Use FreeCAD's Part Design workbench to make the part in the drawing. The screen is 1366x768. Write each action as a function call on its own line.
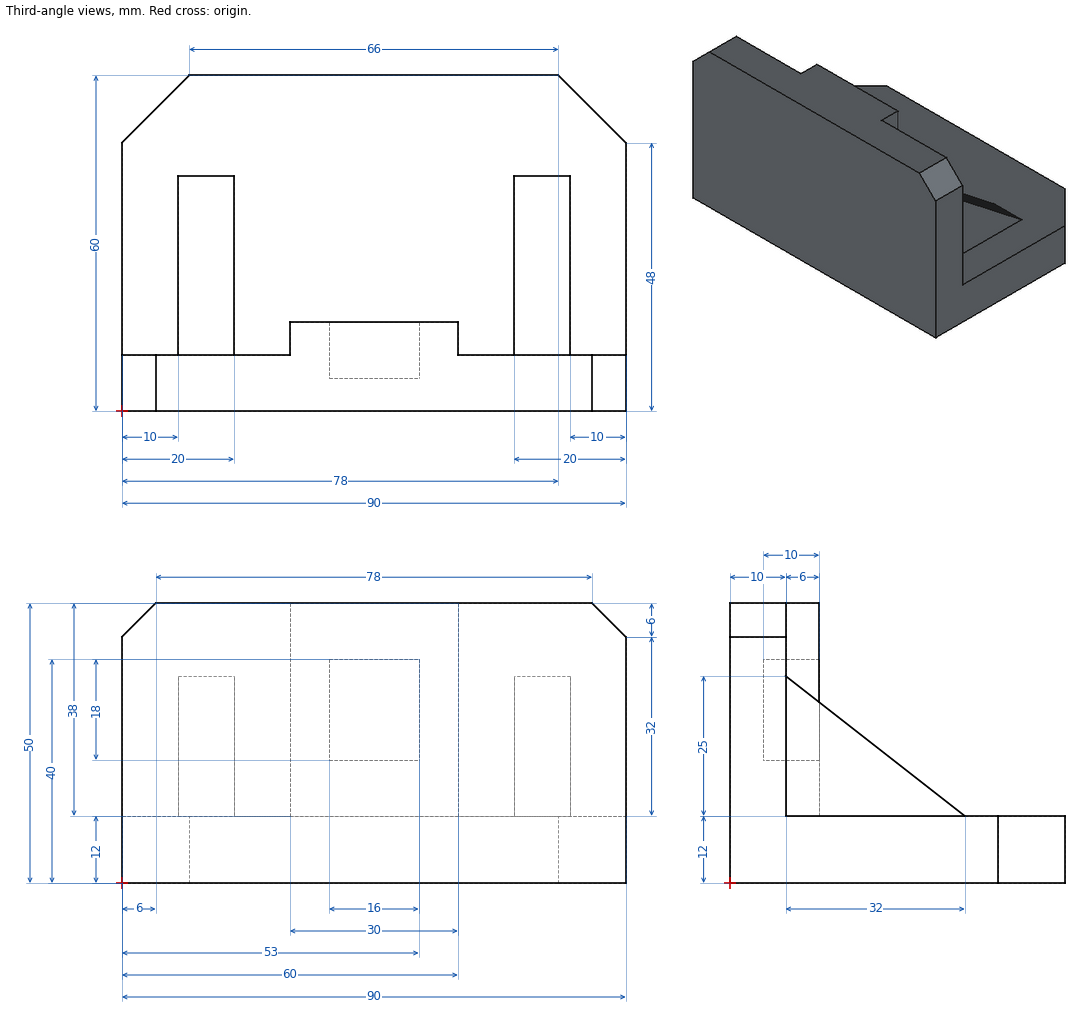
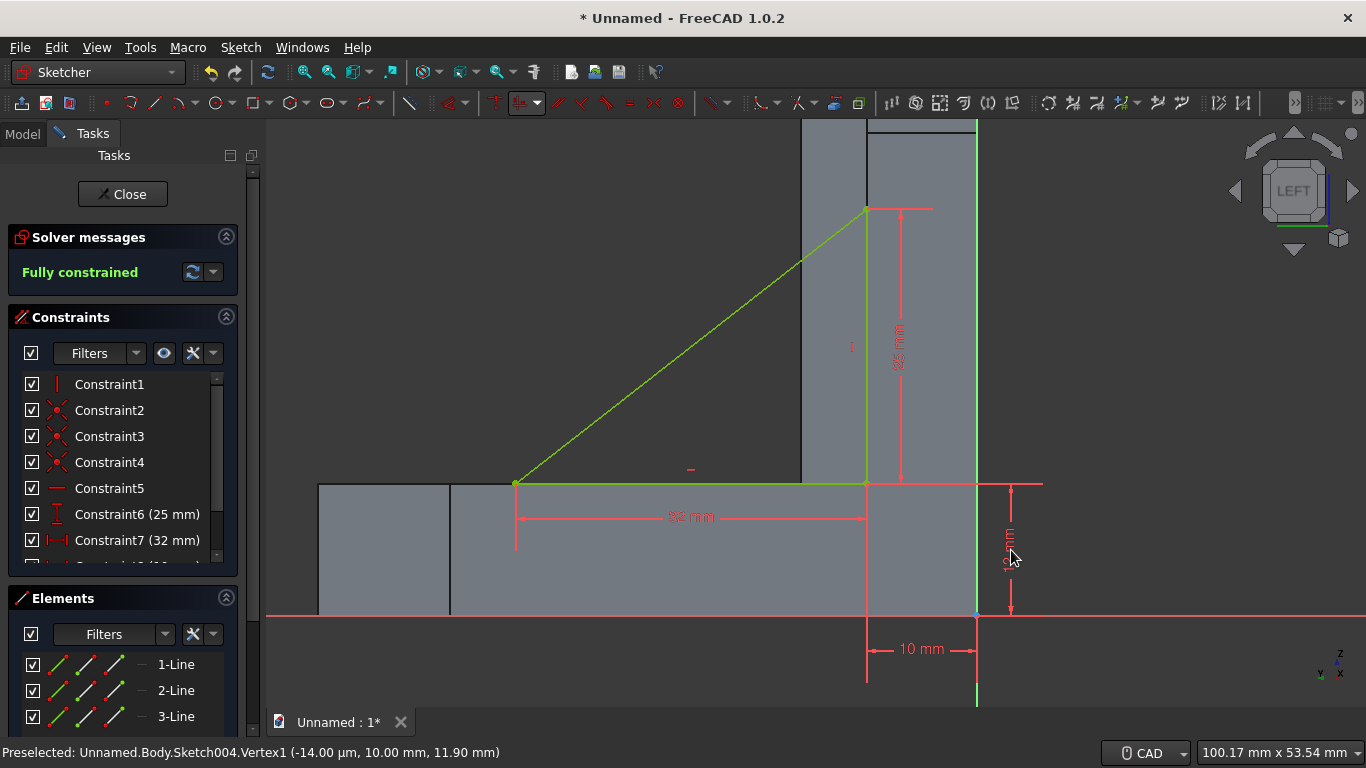
click(123, 194)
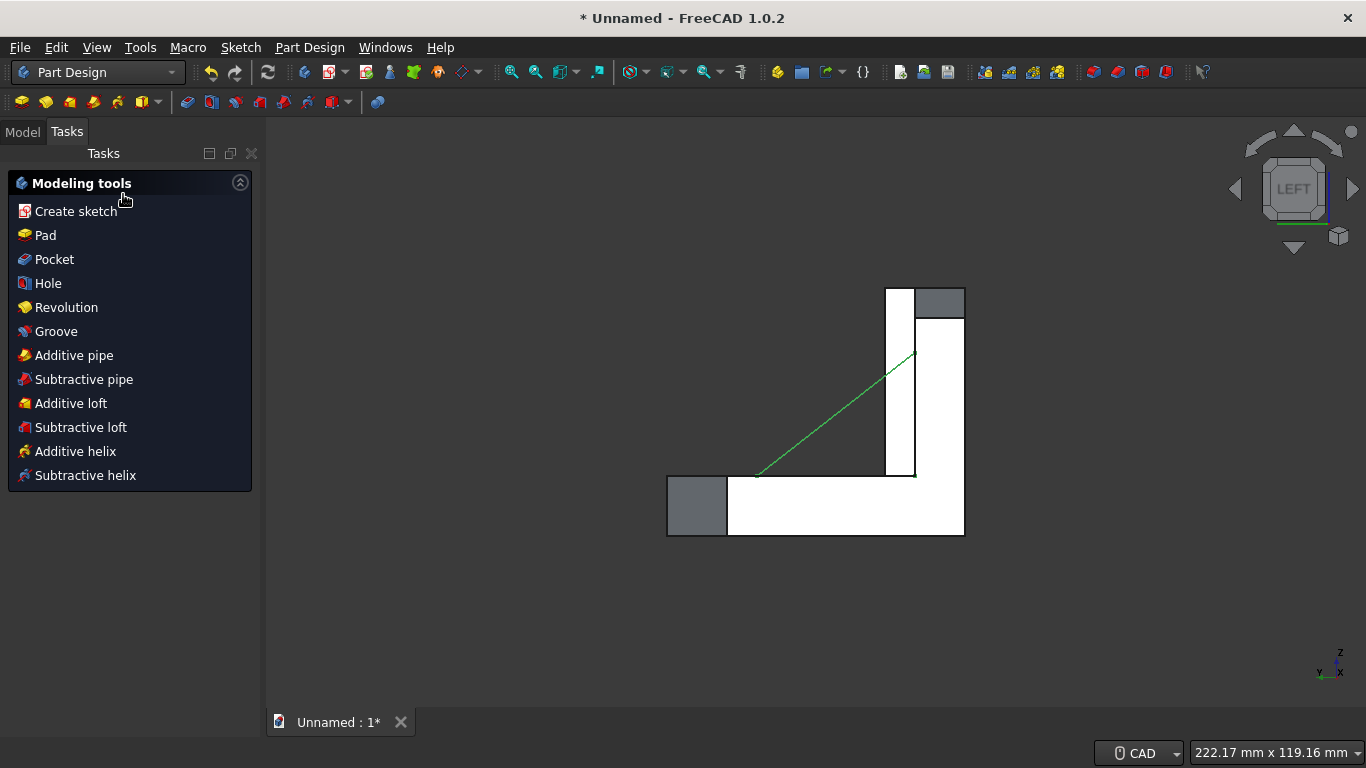
click(22, 102)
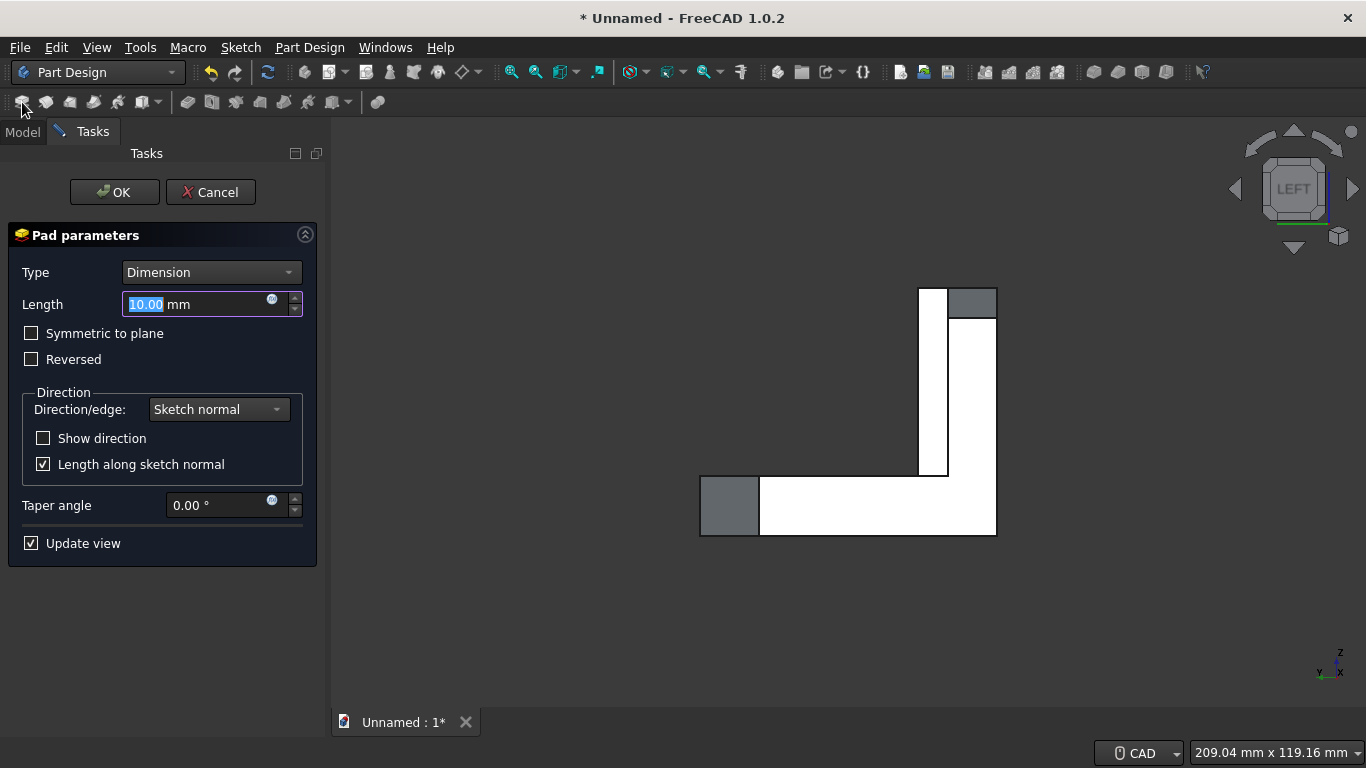
text(20)
key(Tab)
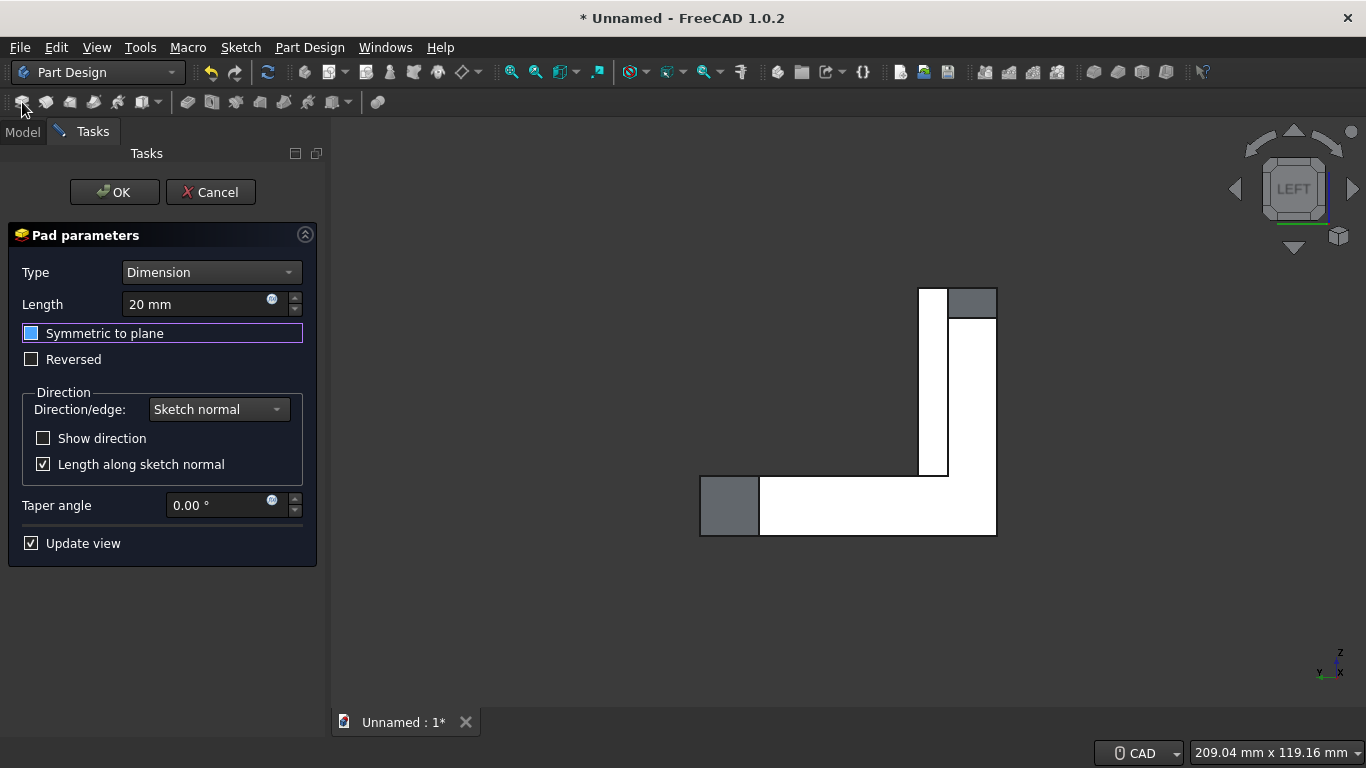
click(30, 359)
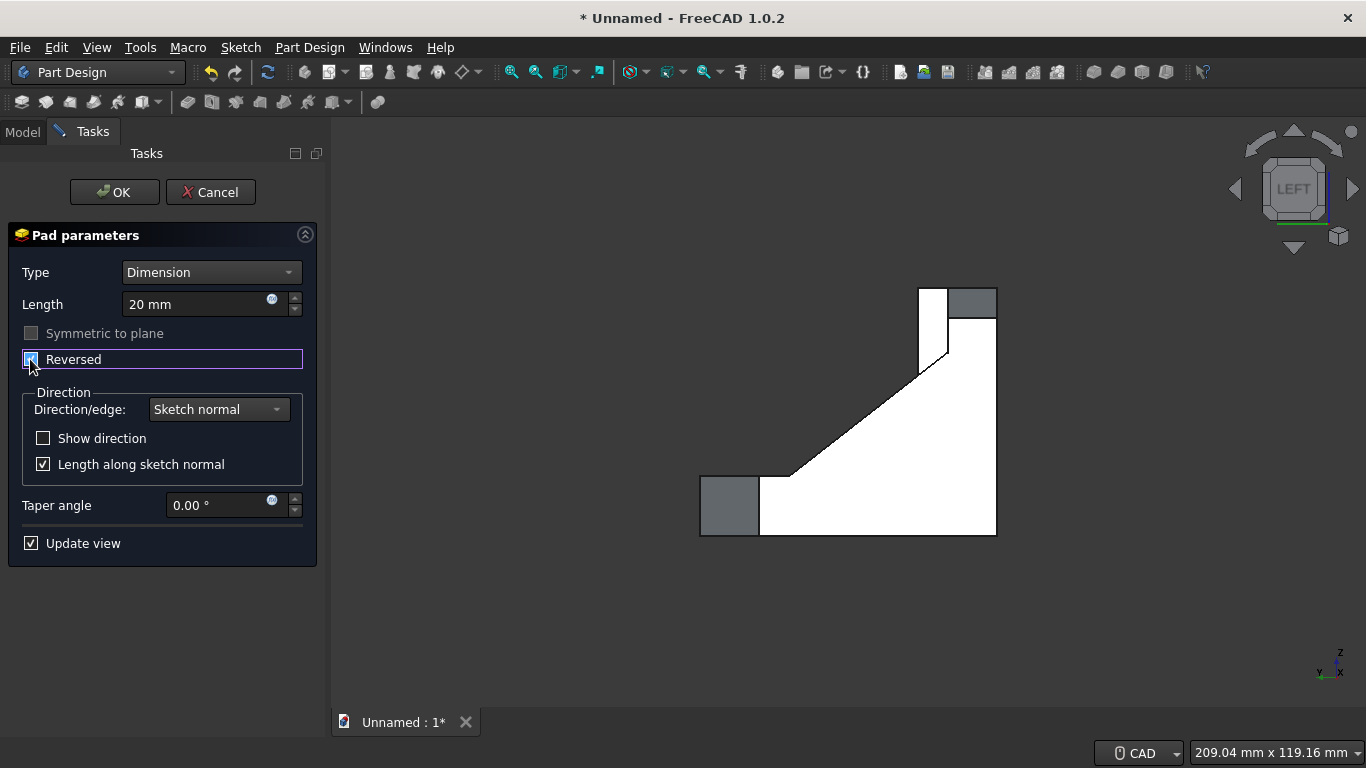
click(115, 192)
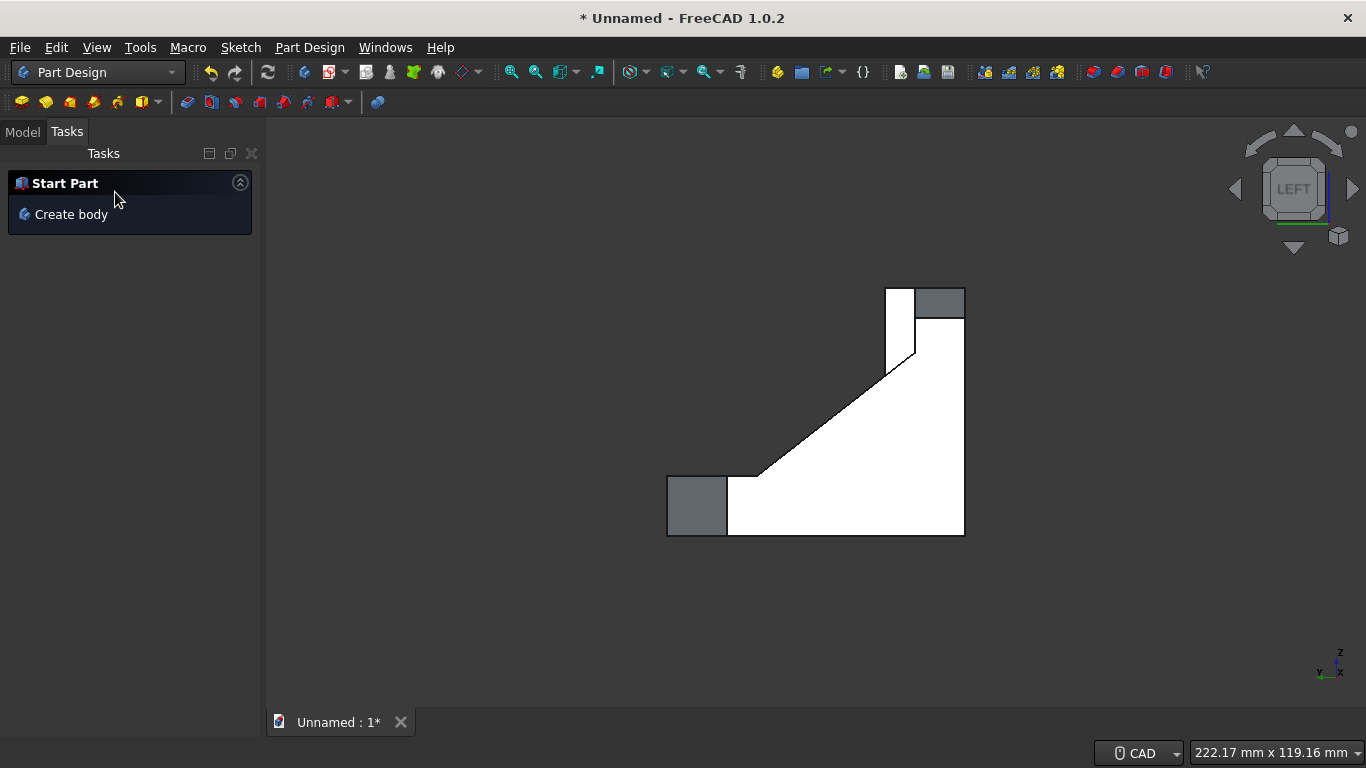
click(512, 72)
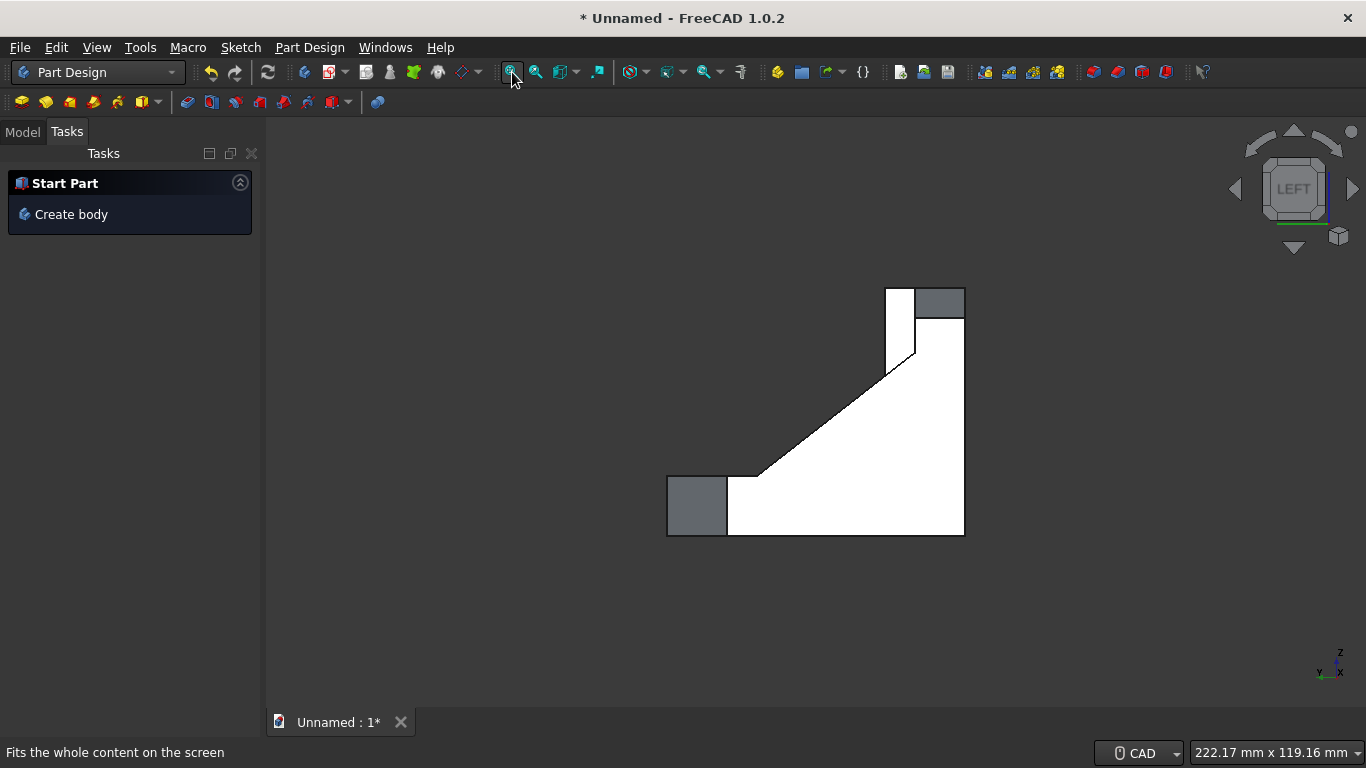
key(0)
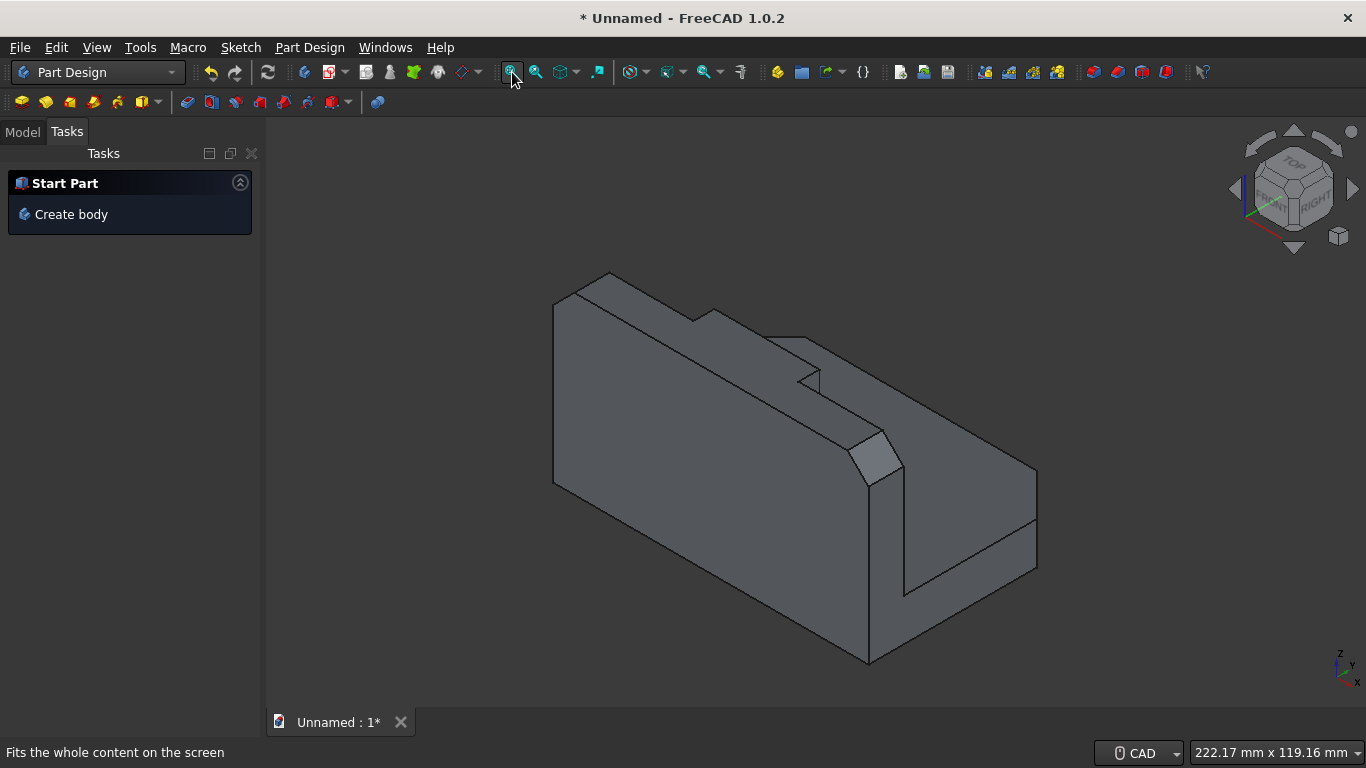
click(881, 517)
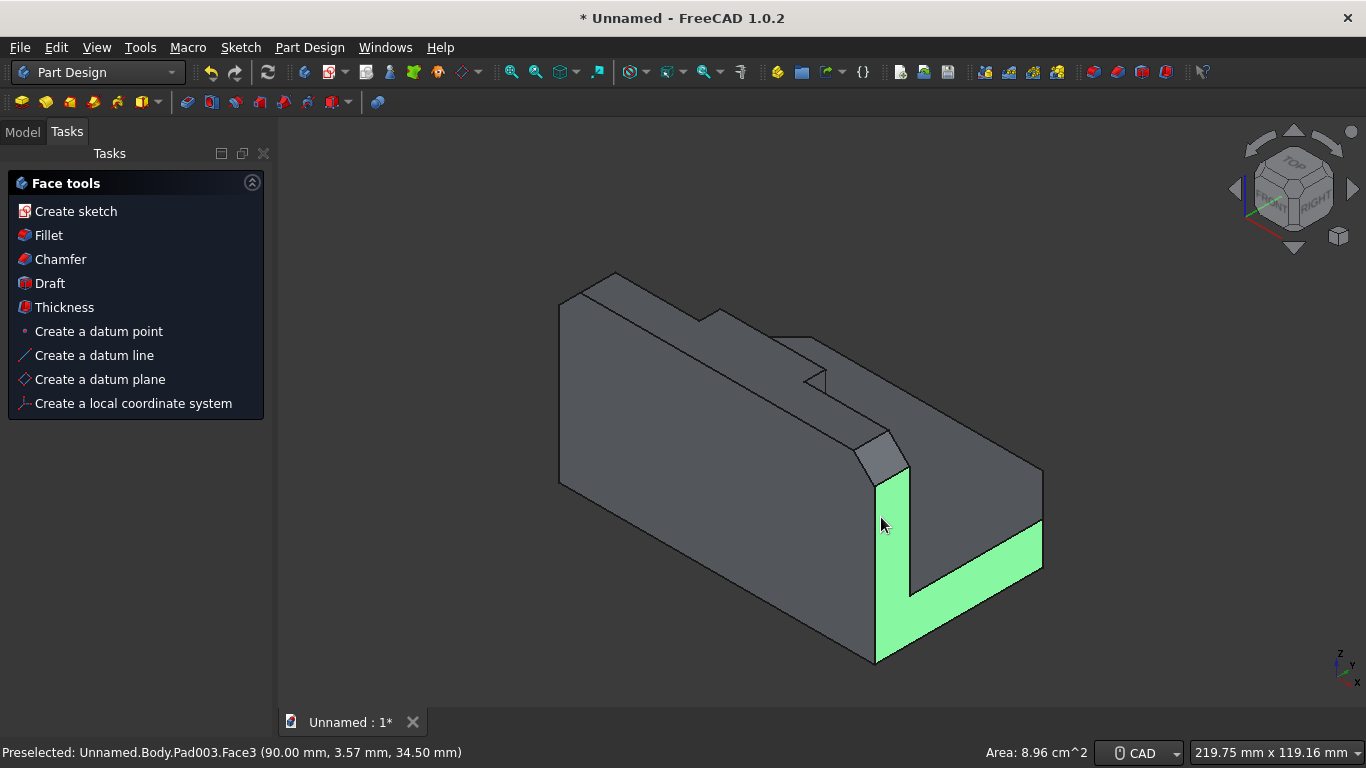
click(330, 72)